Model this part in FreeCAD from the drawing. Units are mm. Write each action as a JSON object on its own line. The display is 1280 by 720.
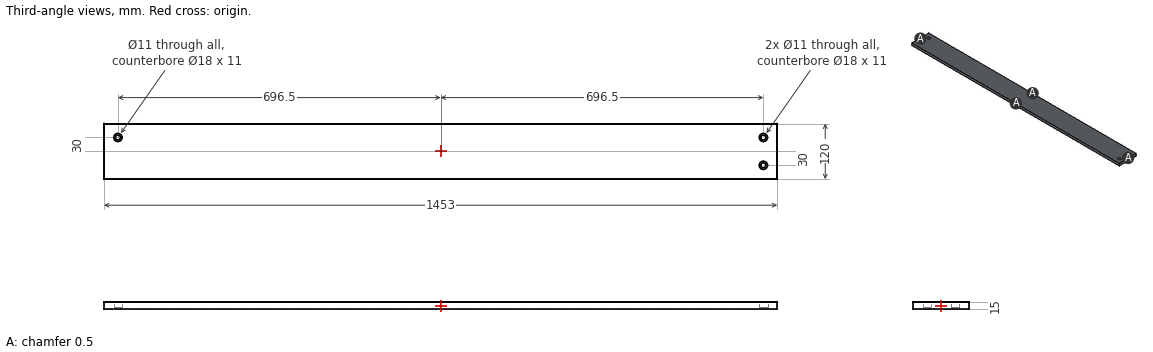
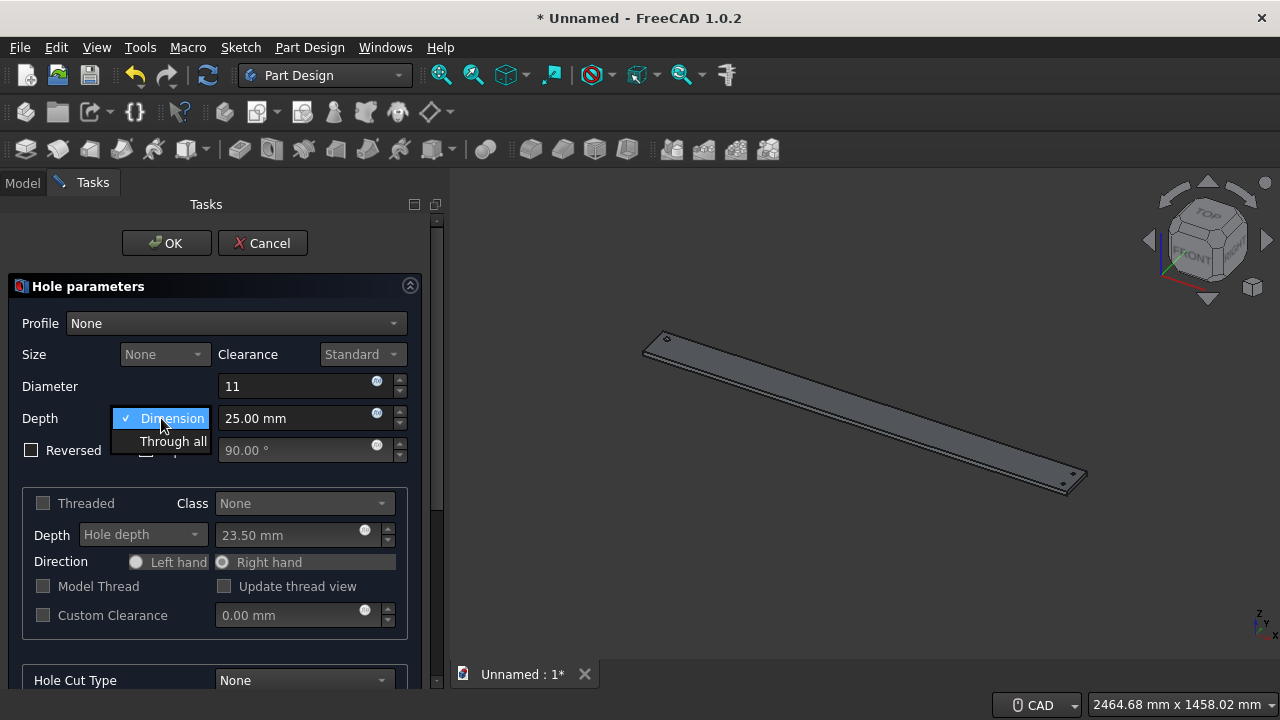
{"action": "left_click", "coordinate": [160, 442]}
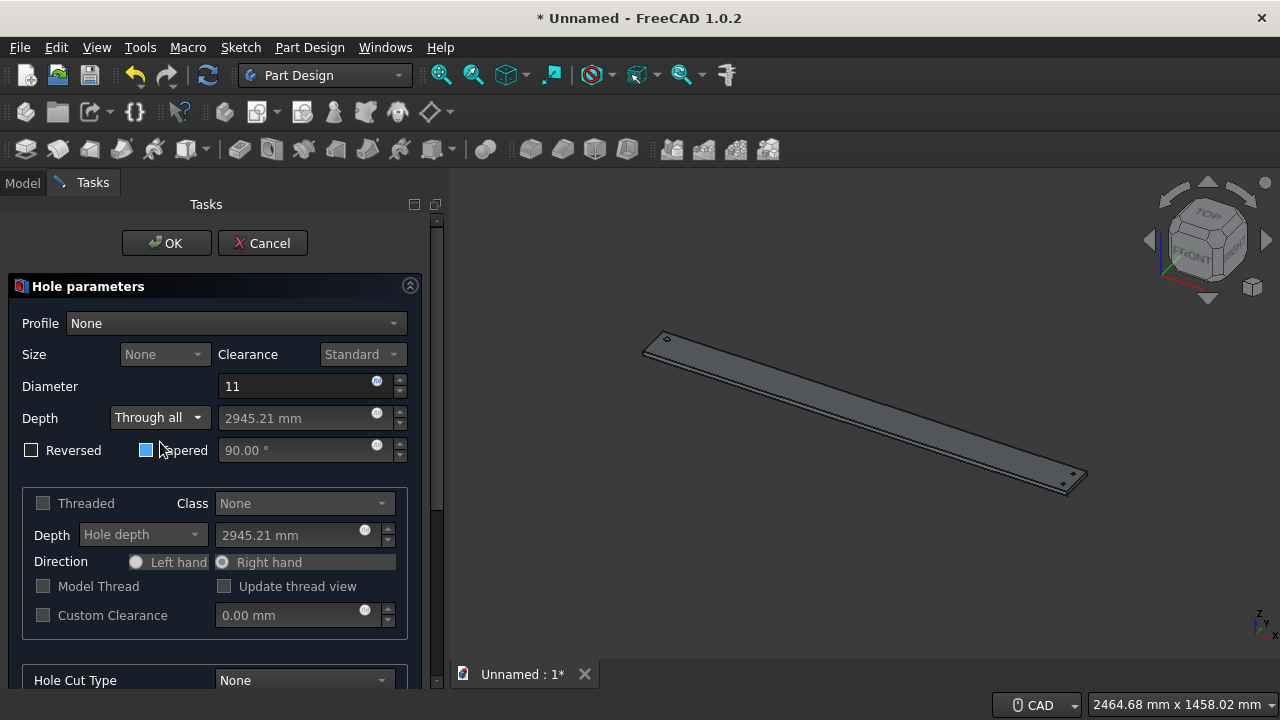
{"action": "scroll", "coordinate": [437, 451], "scroll_direction": "down", "scroll_amount": 2}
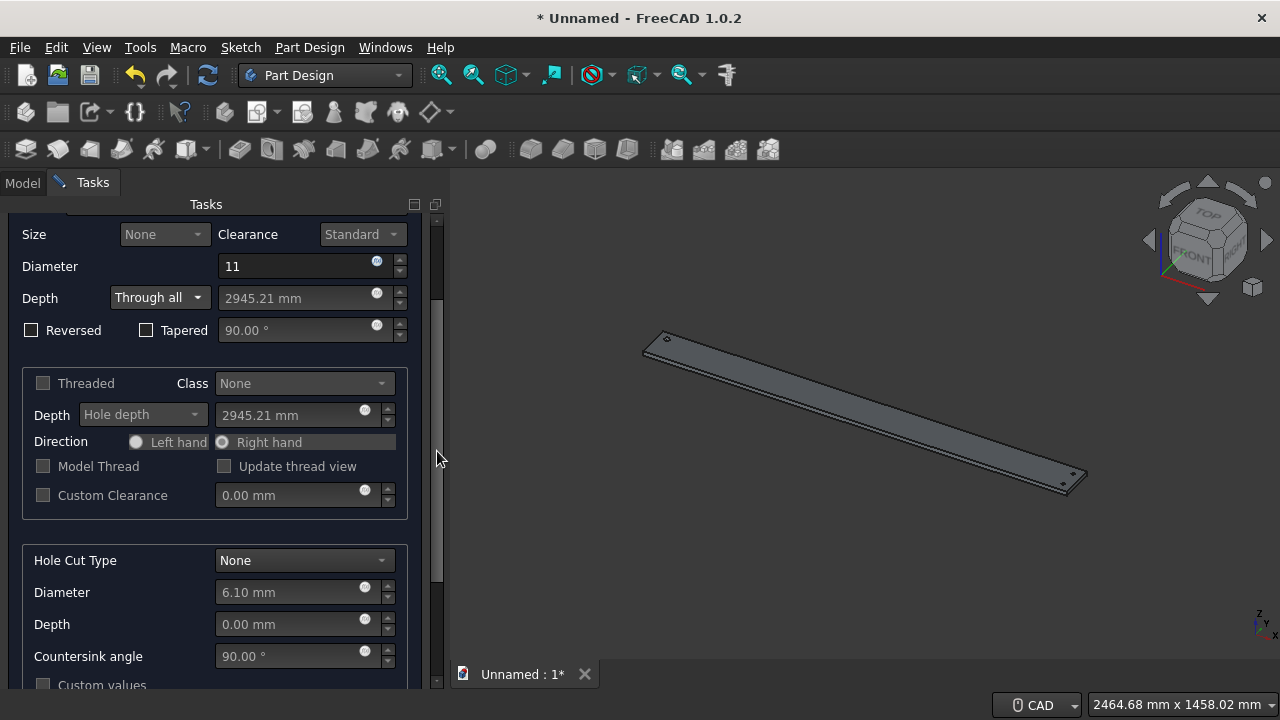
{"action": "left_click", "coordinate": [306, 560]}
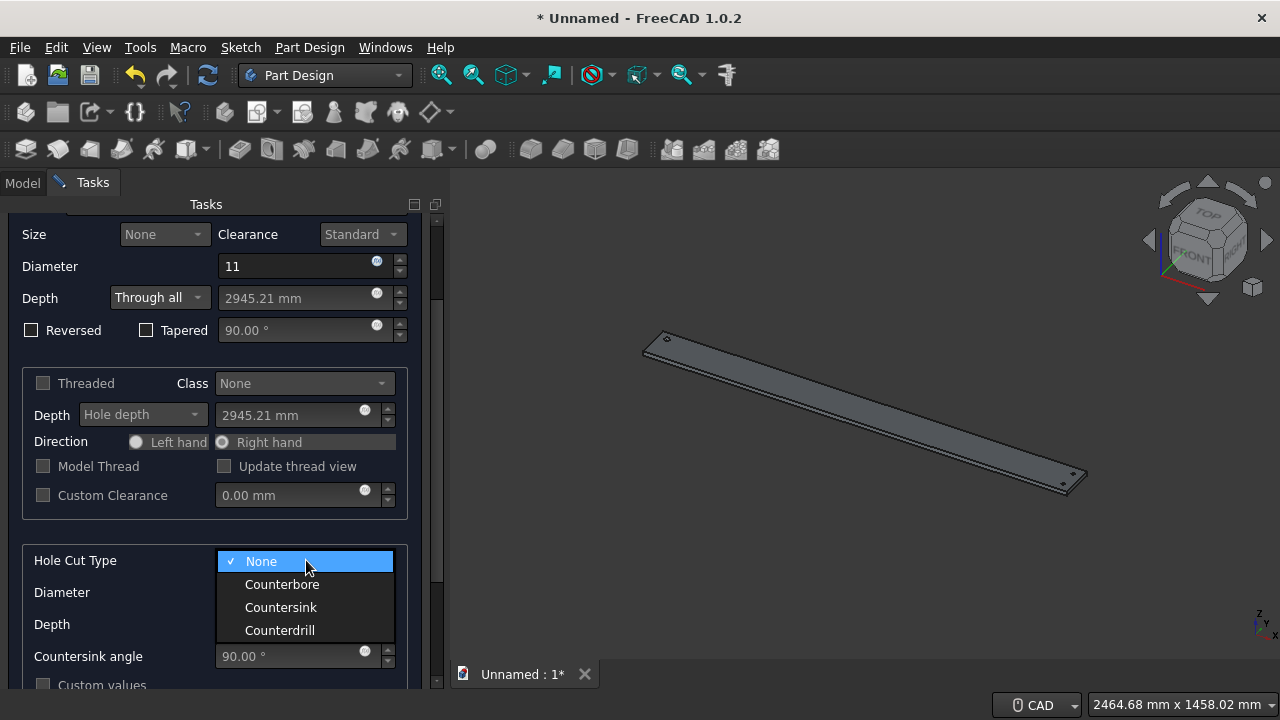
{"action": "left_click", "coordinate": [304, 584]}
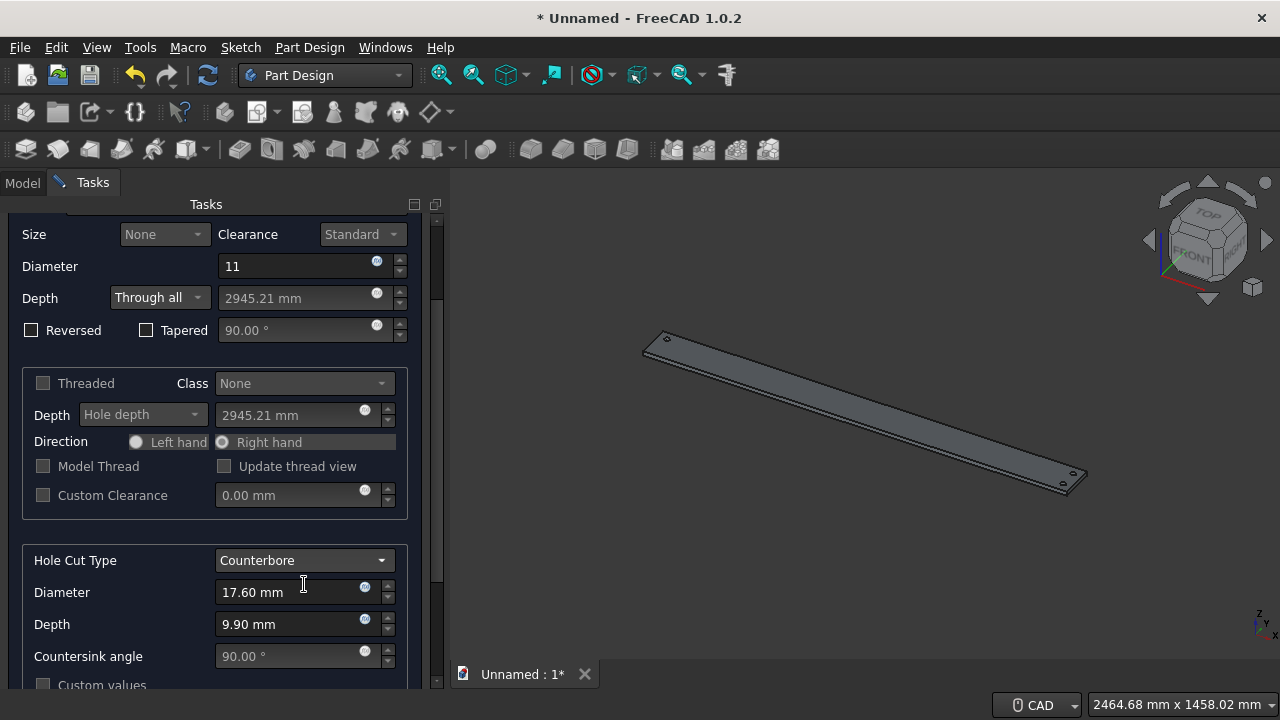
{"action": "triple_click", "coordinate": [298, 592]}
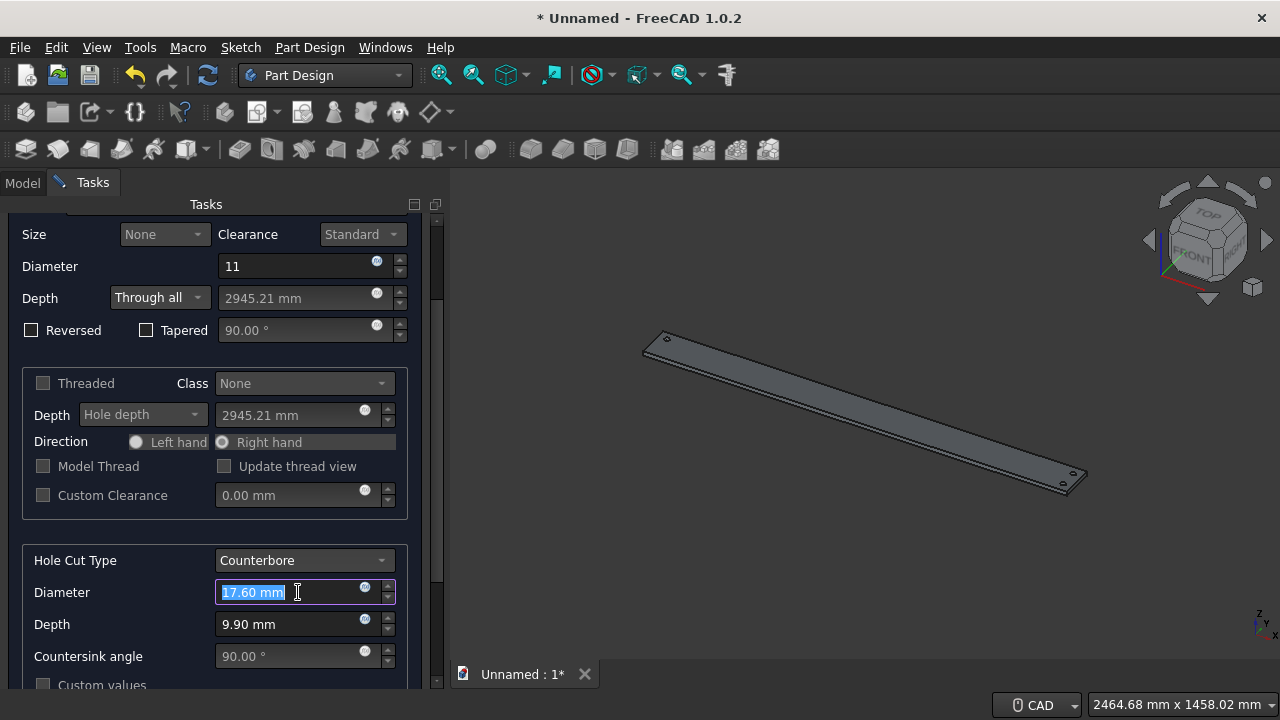
{"action": "type", "text": "18"}
{"action": "key", "text": "Tab"}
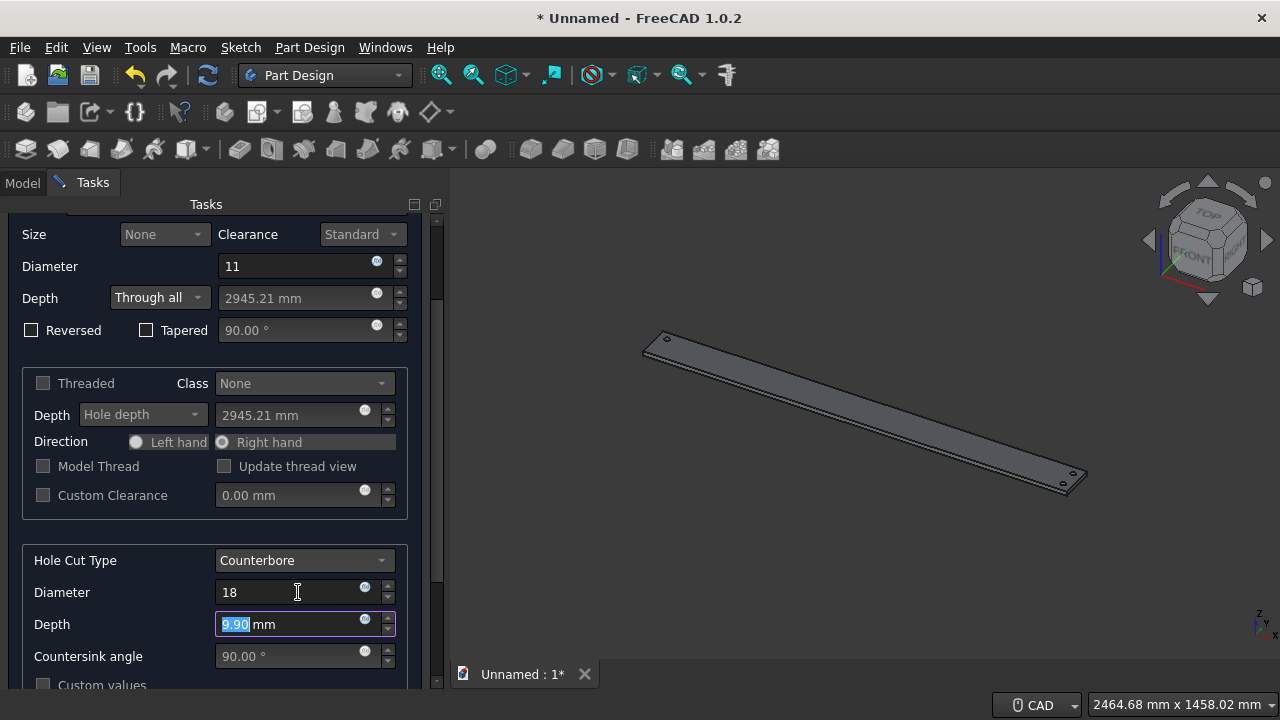
{"action": "type", "text": "11"}
{"action": "key", "text": "Tab"}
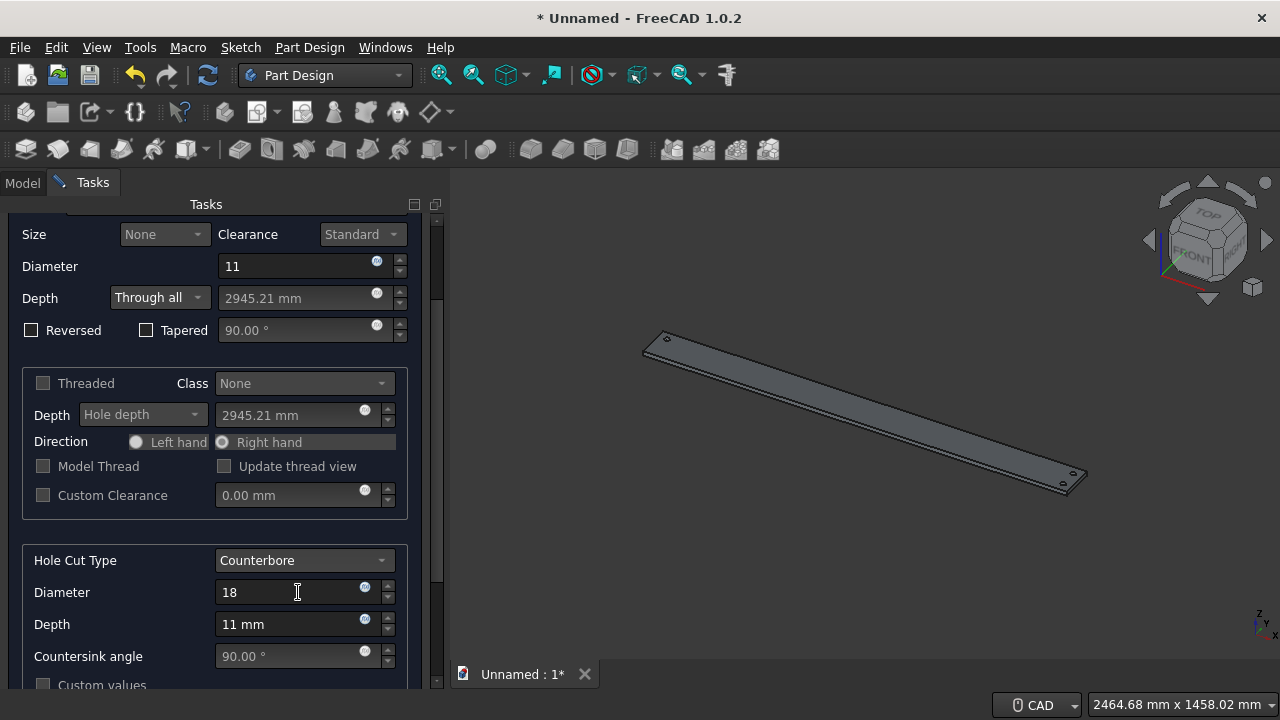
{"action": "scroll", "coordinate": [437, 451], "scroll_direction": "up", "scroll_amount": 3}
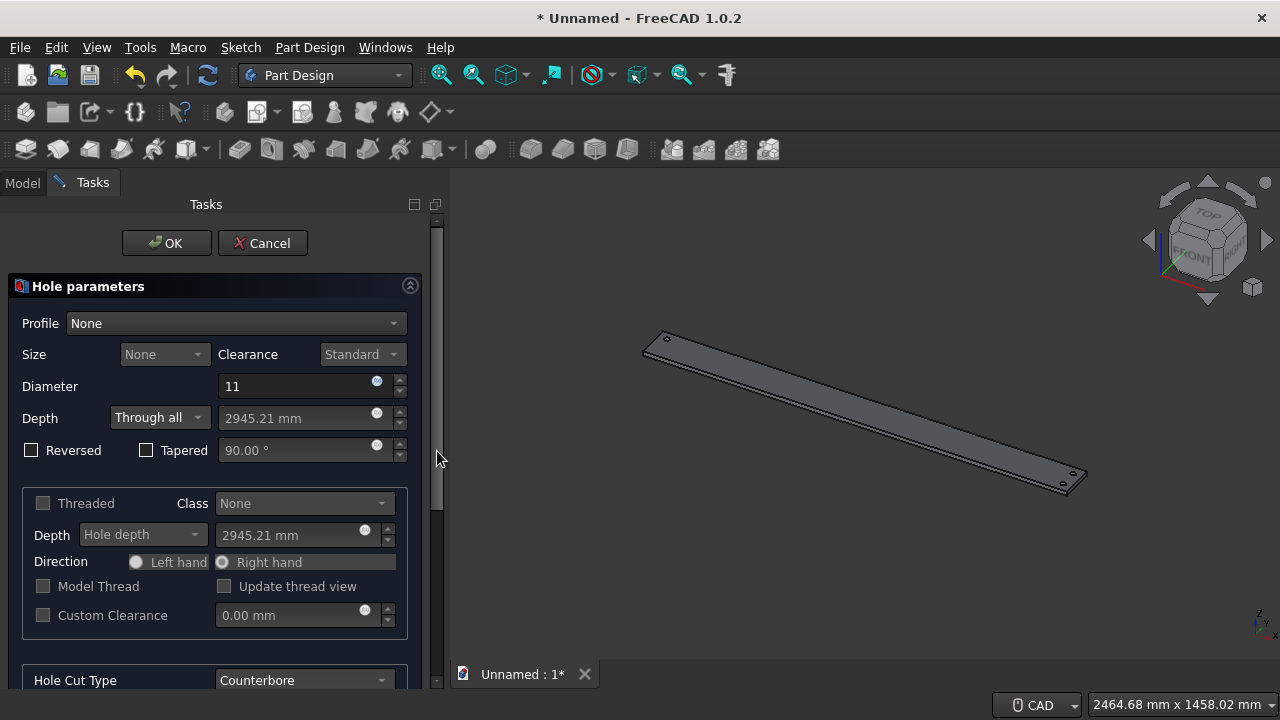
{"action": "left_click", "coordinate": [167, 243]}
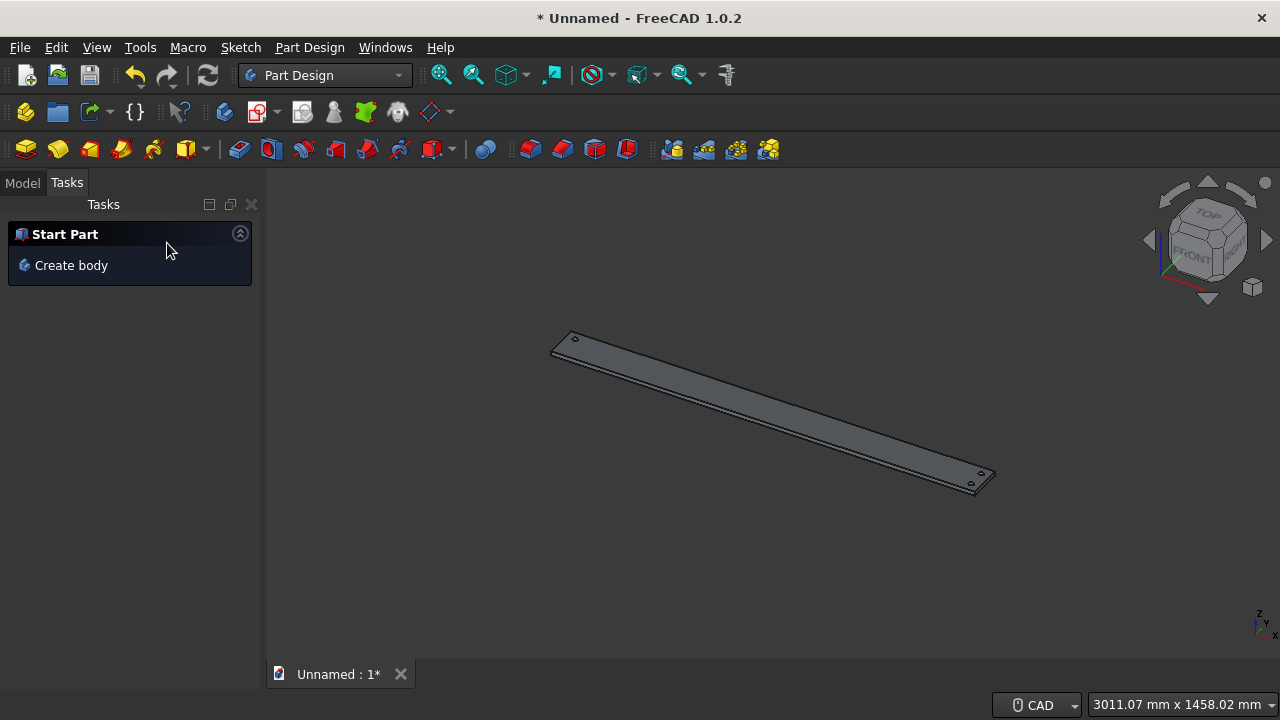
{"action": "left_click", "coordinate": [442, 76]}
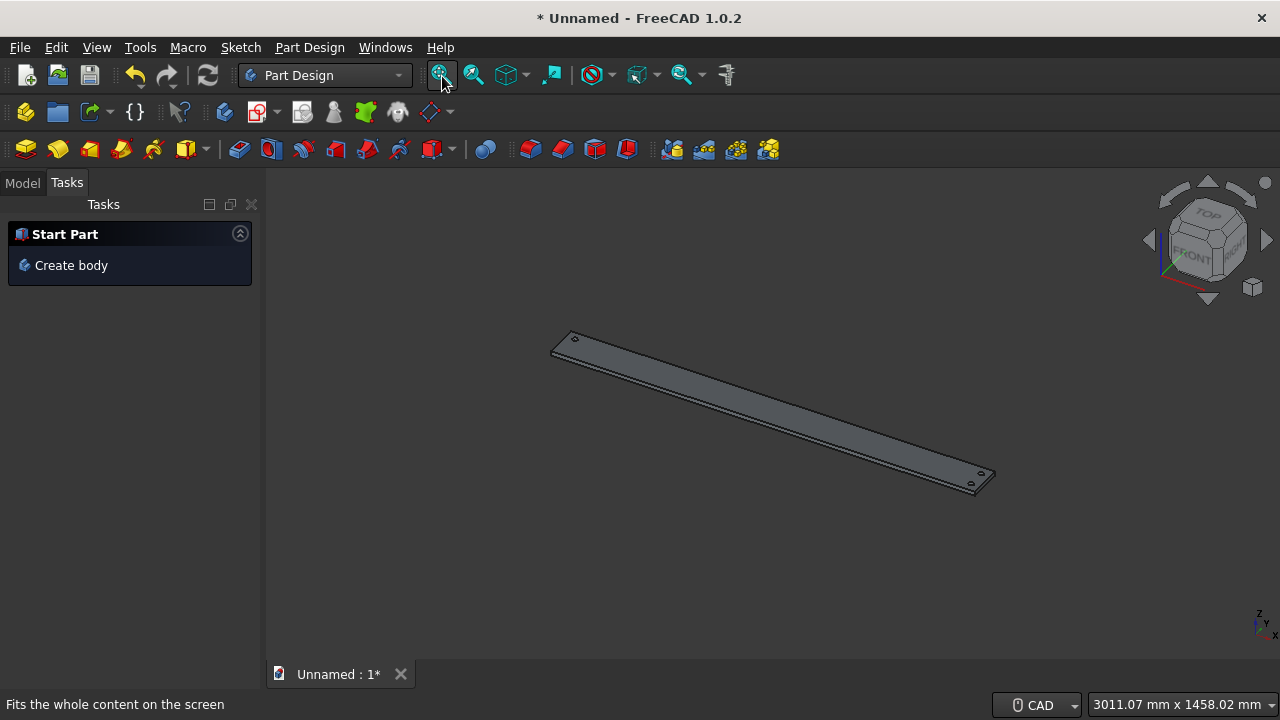
{"action": "left_click", "coordinate": [763, 420]}